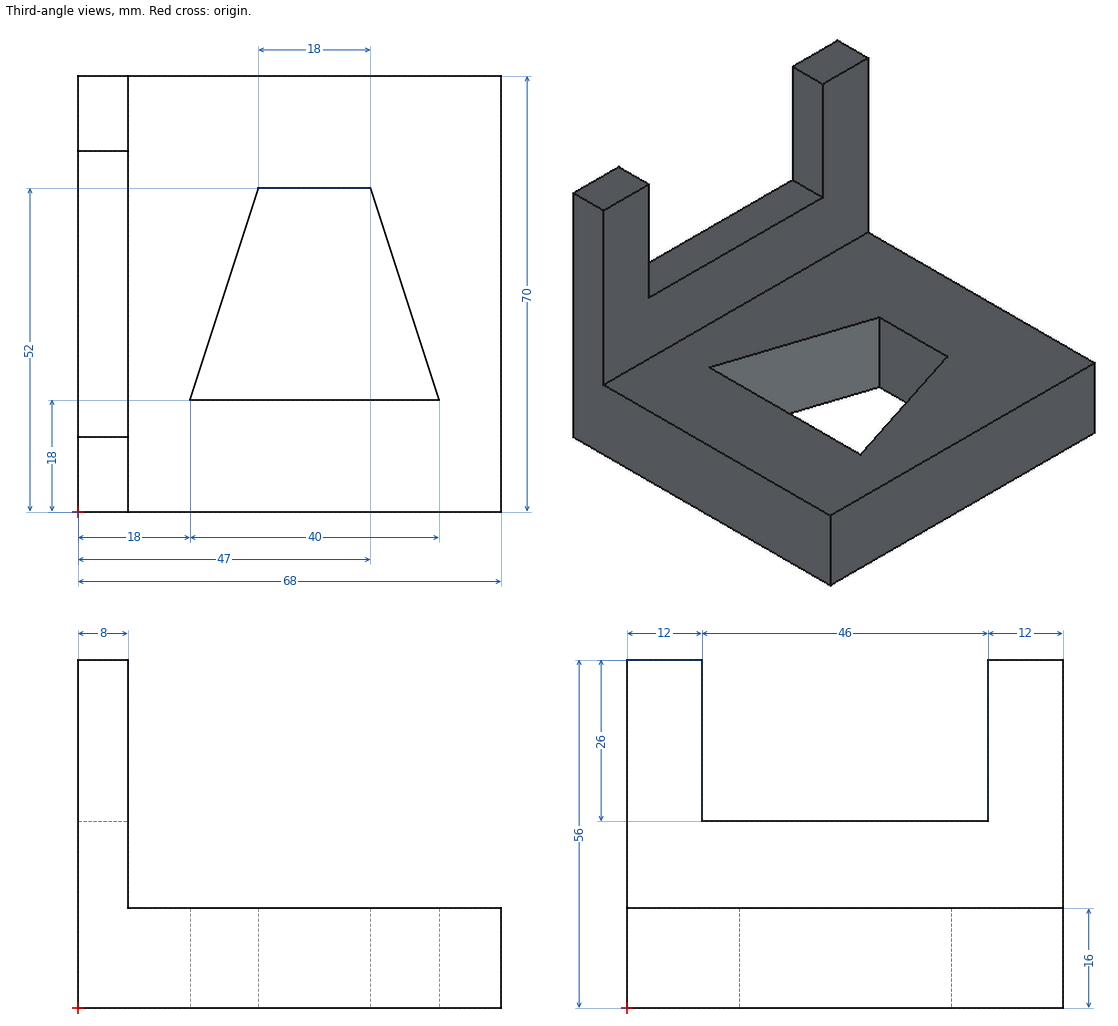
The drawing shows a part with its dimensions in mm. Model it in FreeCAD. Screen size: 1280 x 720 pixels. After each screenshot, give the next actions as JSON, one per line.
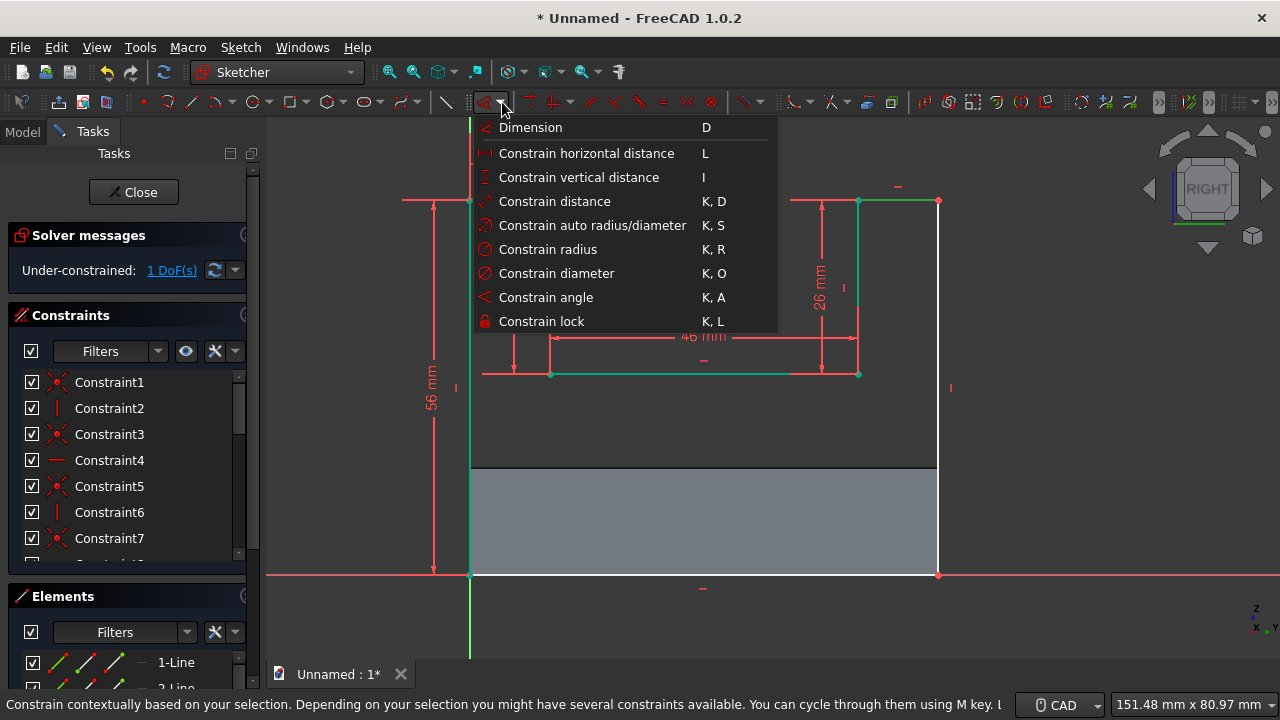
{"action": "left_click", "coordinate": [626, 153]}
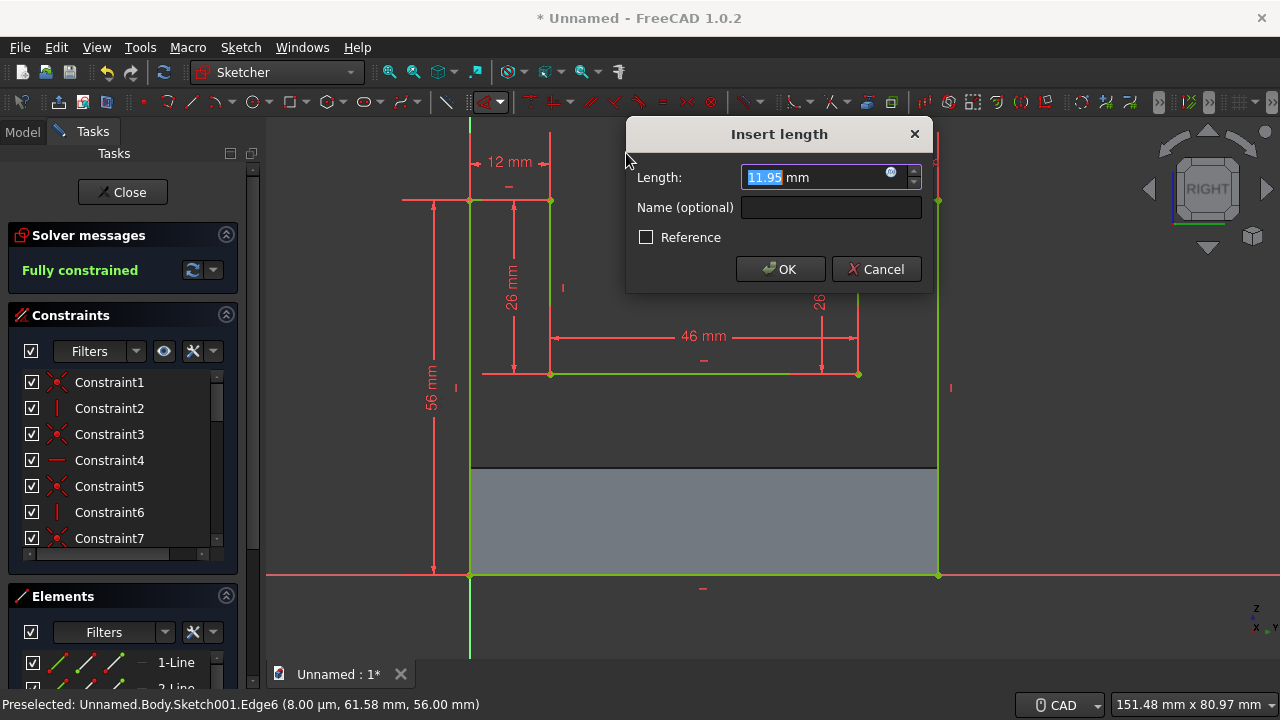
{"action": "type", "text": "12"}
{"action": "key", "text": "Return"}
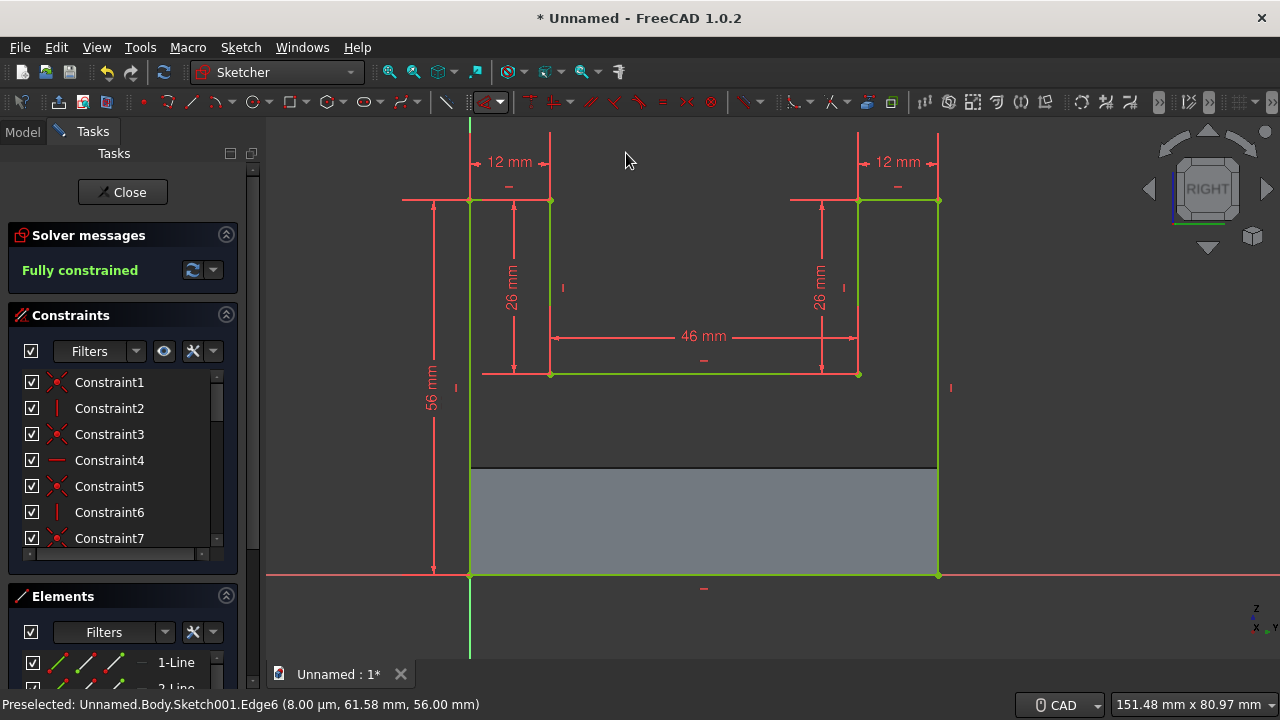
{"action": "left_click", "coordinate": [123, 192]}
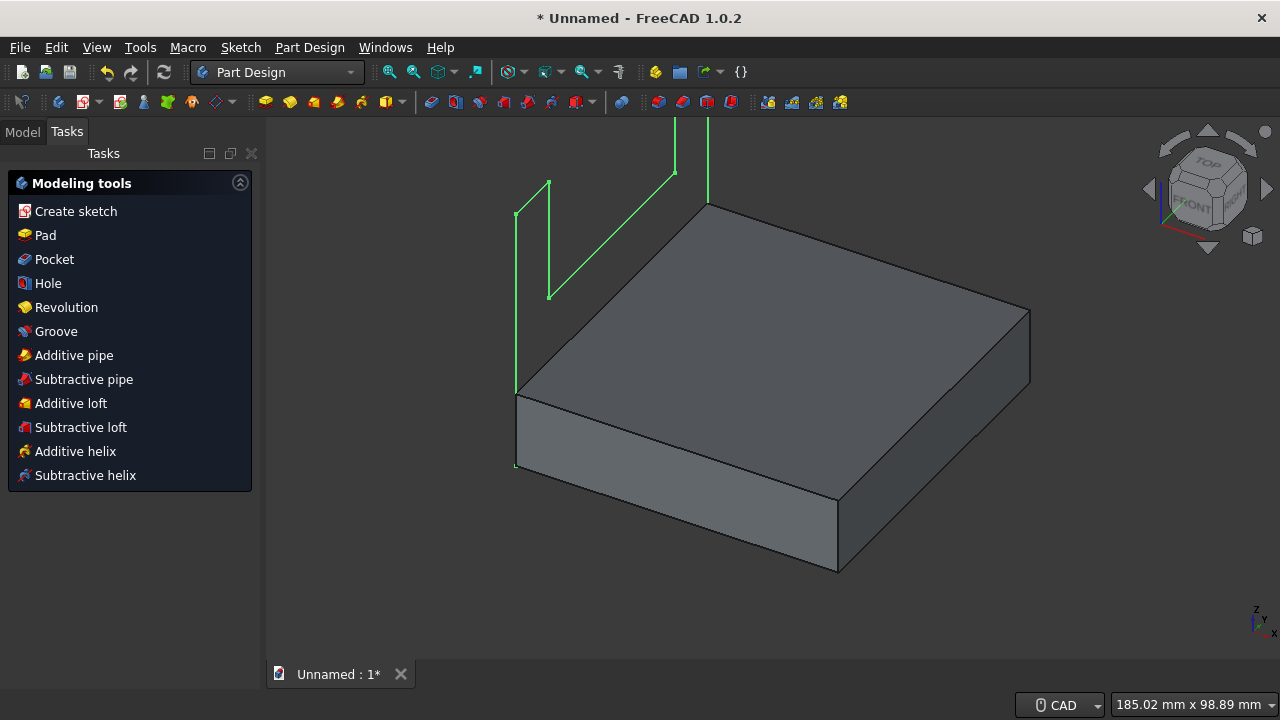
{"action": "left_click", "coordinate": [266, 102]}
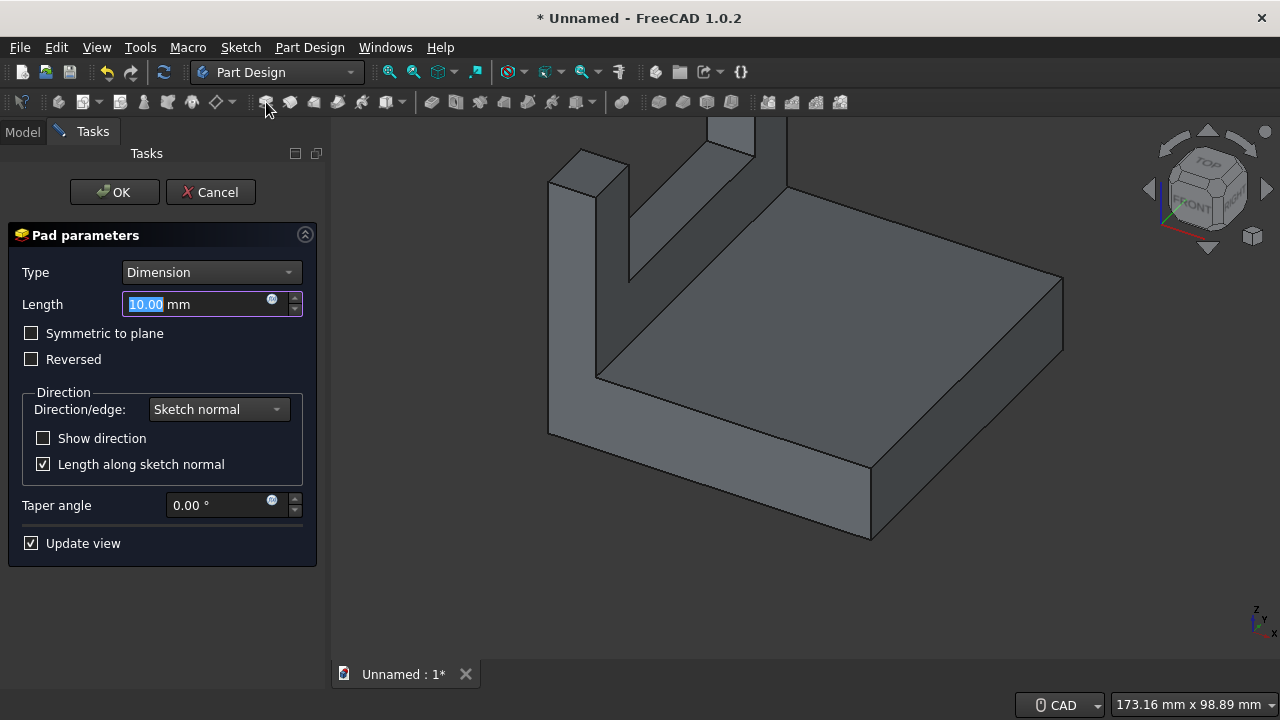
{"action": "type", "text": "8"}
{"action": "key", "text": "Tab"}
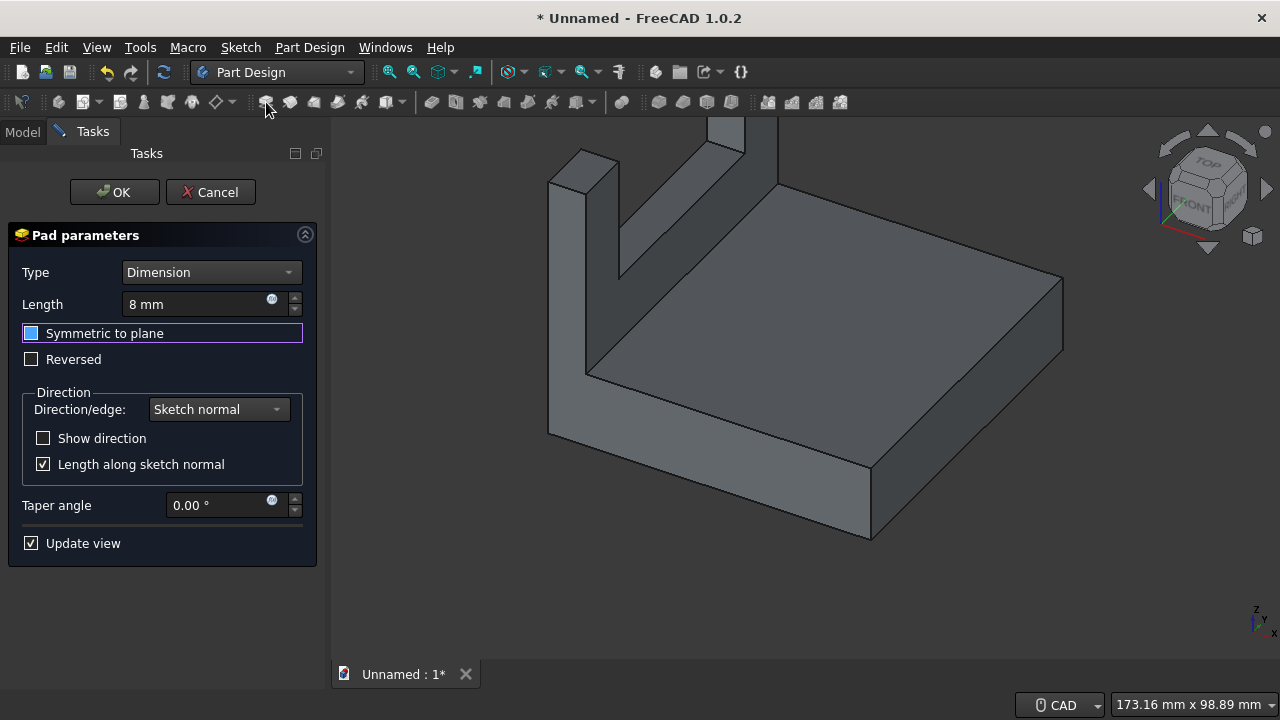
{"action": "left_click", "coordinate": [115, 192]}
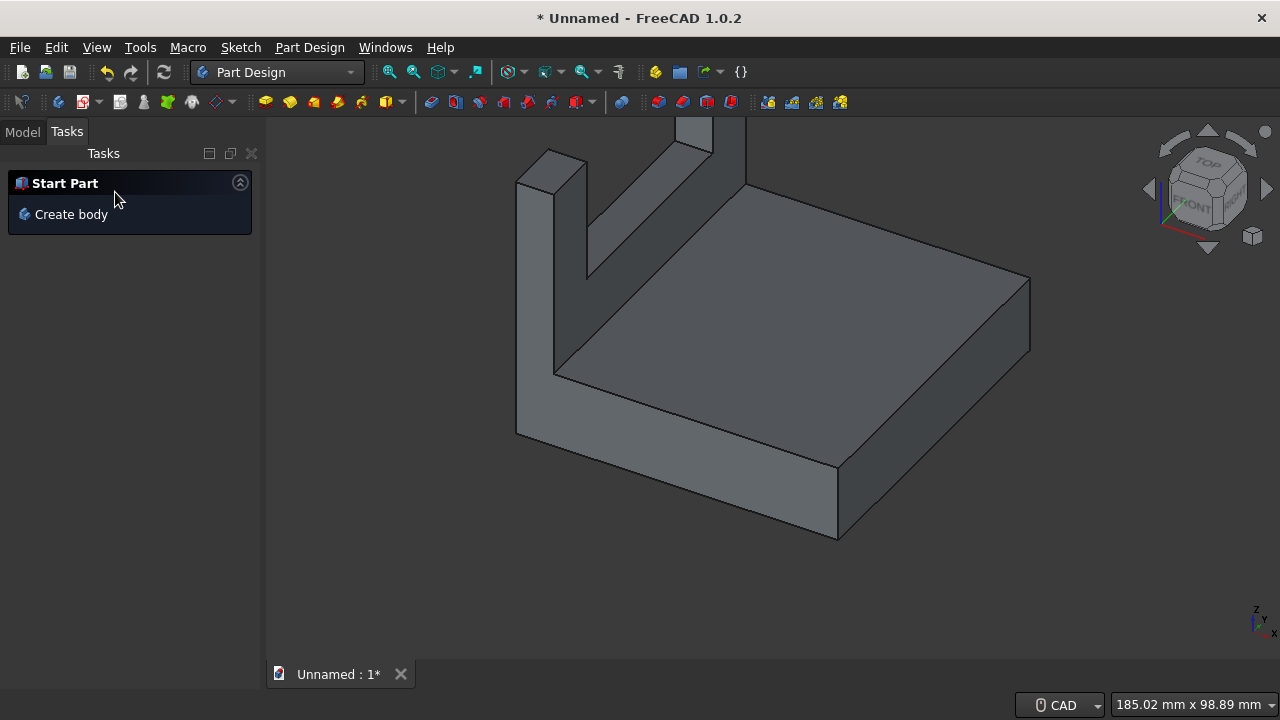
{"action": "key", "text": "v f"}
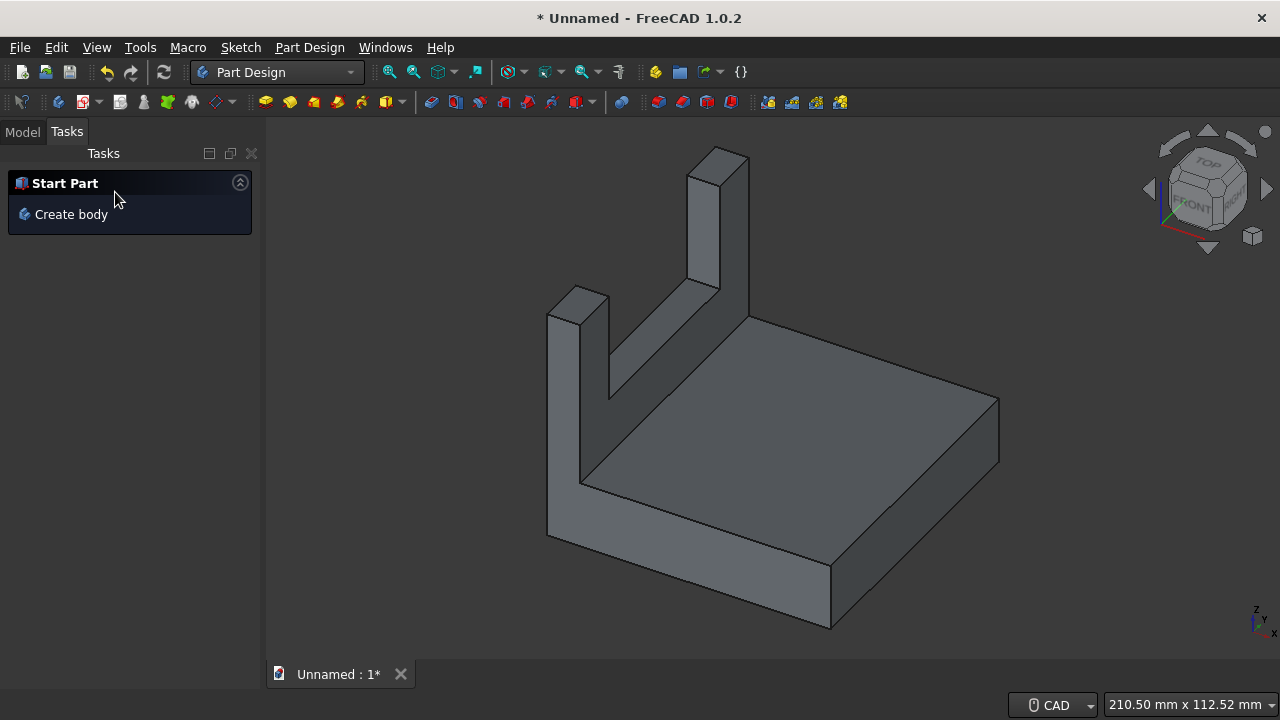
{"action": "left_click", "coordinate": [790, 440]}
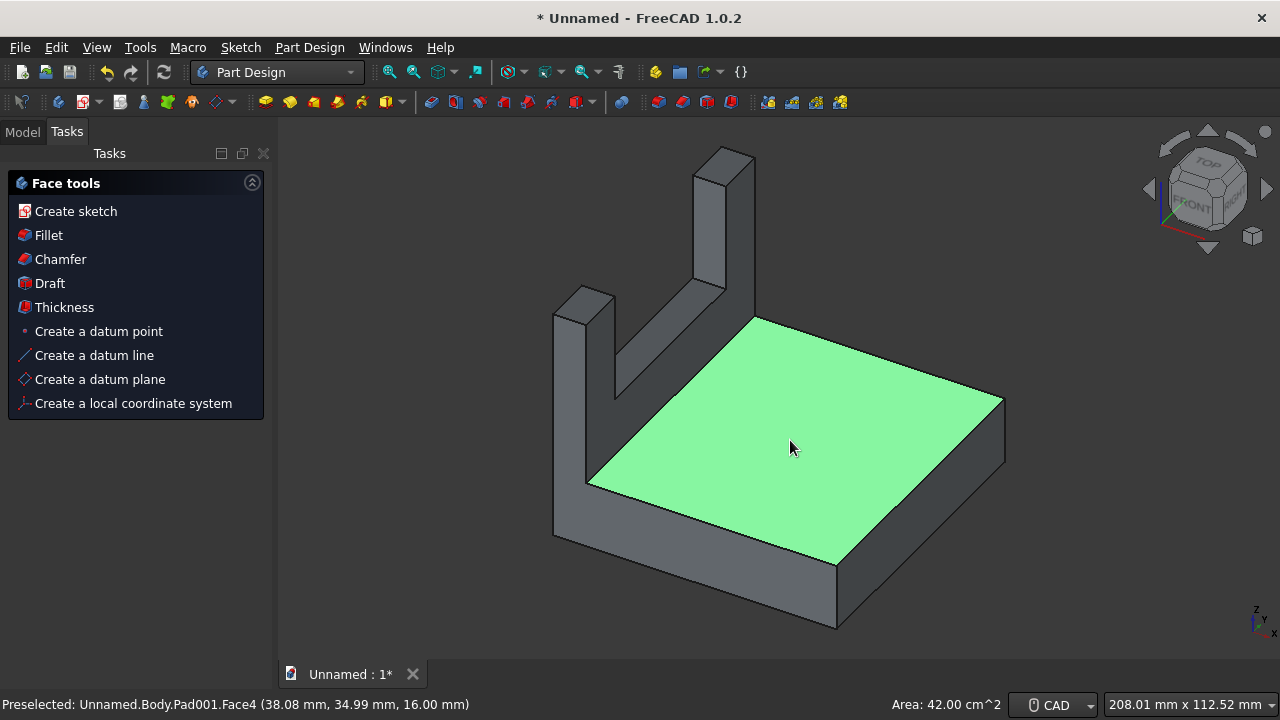
{"action": "left_click", "coordinate": [84, 102]}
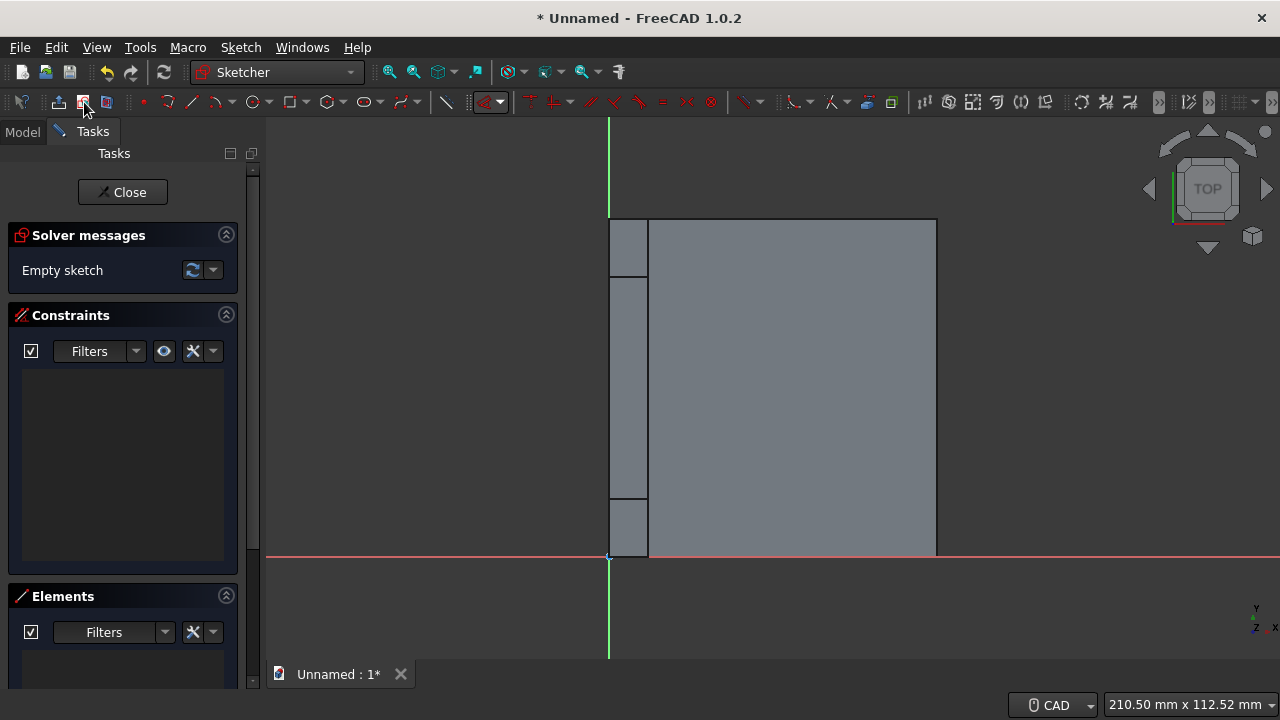
{"action": "key", "text": "q s"}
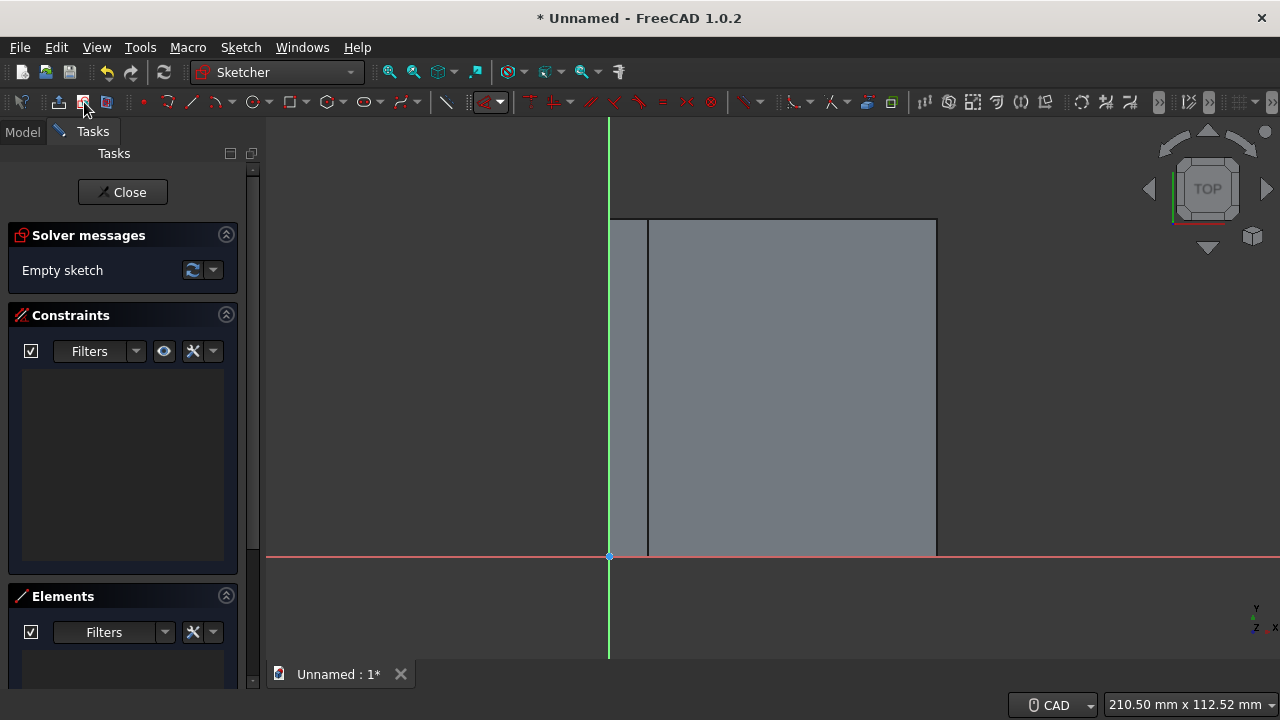
{"action": "scroll", "coordinate": [839, 520], "scroll_direction": "up", "scroll_amount": 2}